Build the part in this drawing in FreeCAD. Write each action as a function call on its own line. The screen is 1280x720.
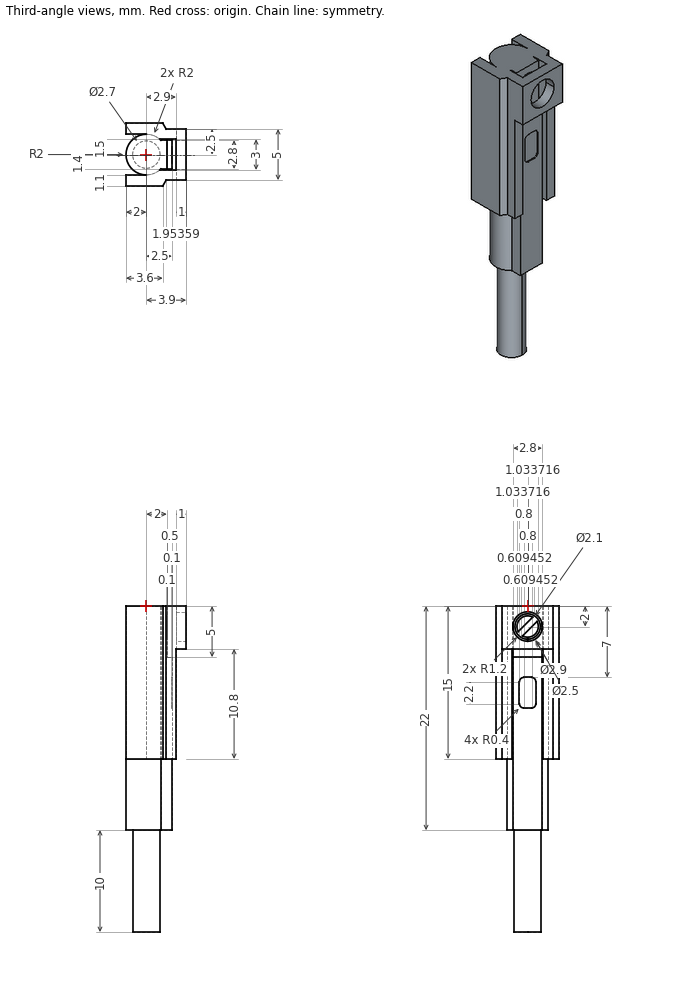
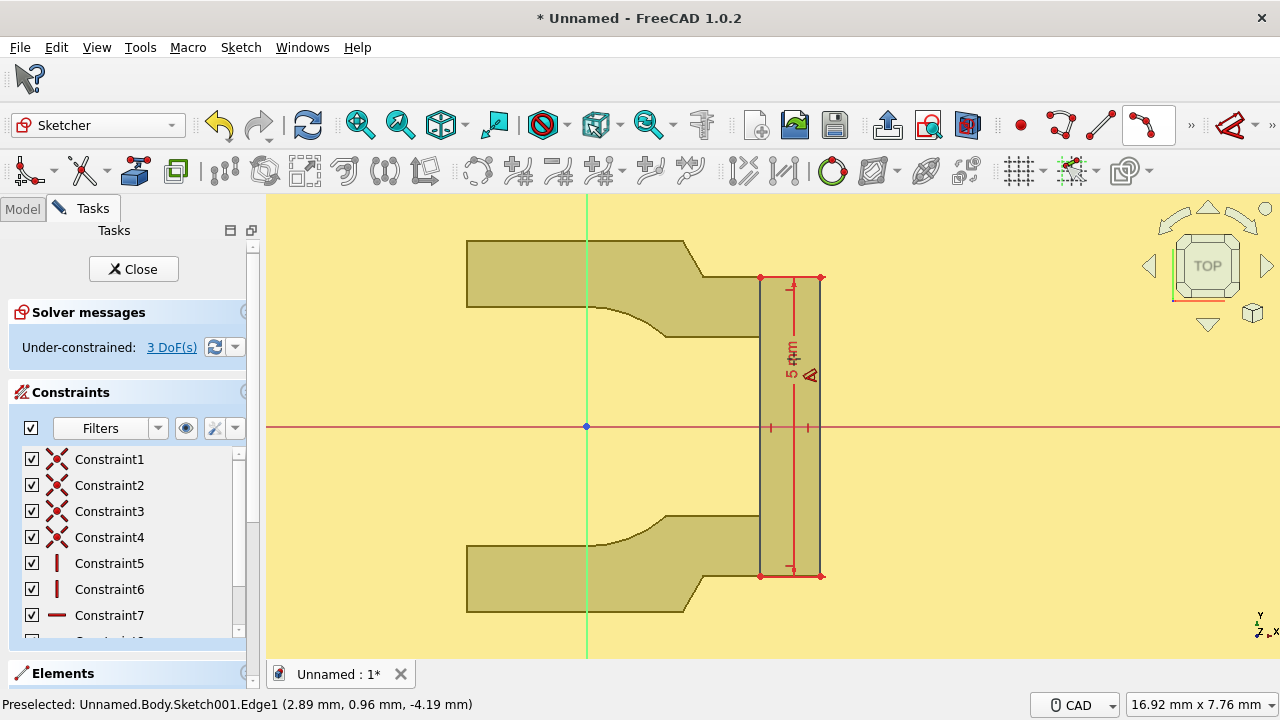
click(778, 577)
click(790, 611)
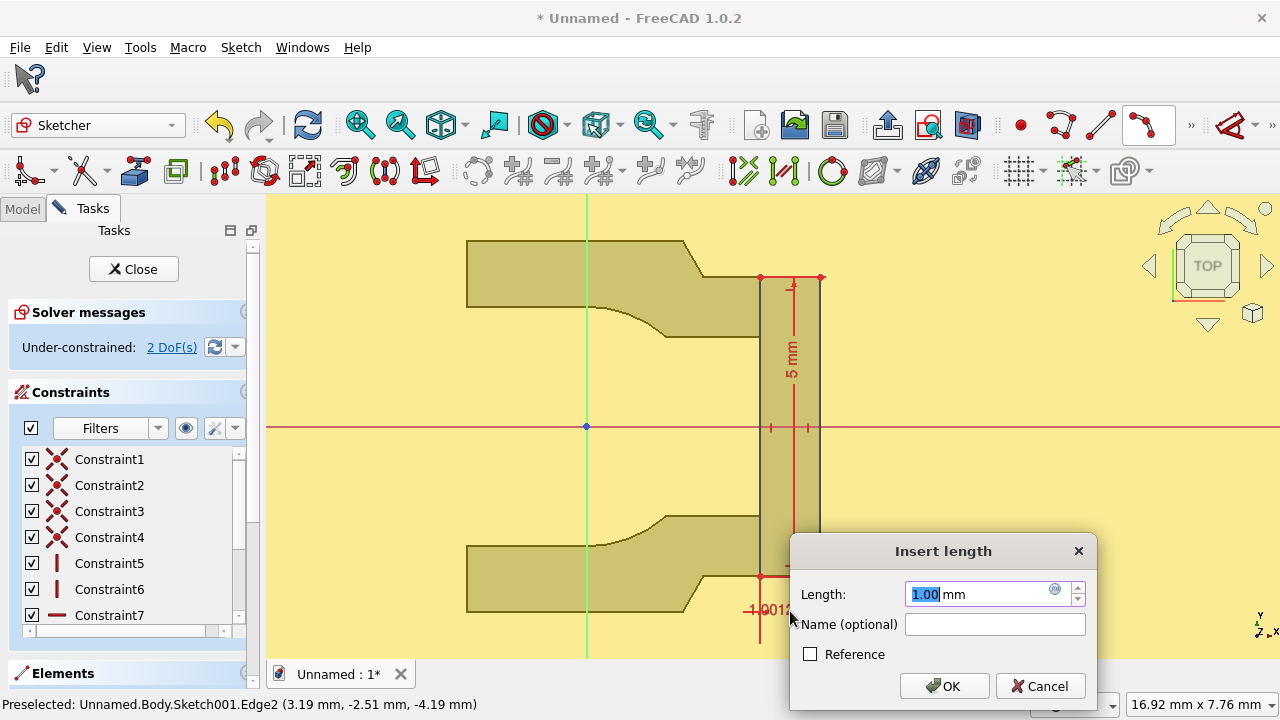
text(1)
key(Return)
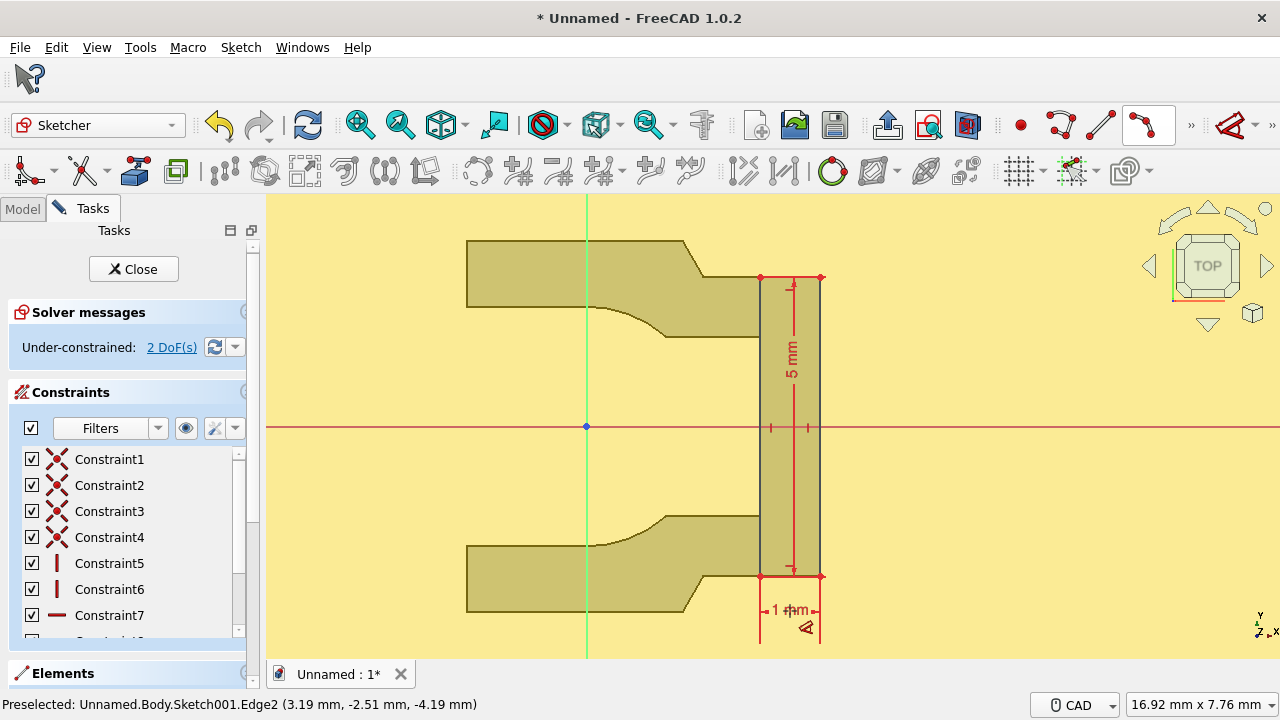
click(760, 277)
click(673, 243)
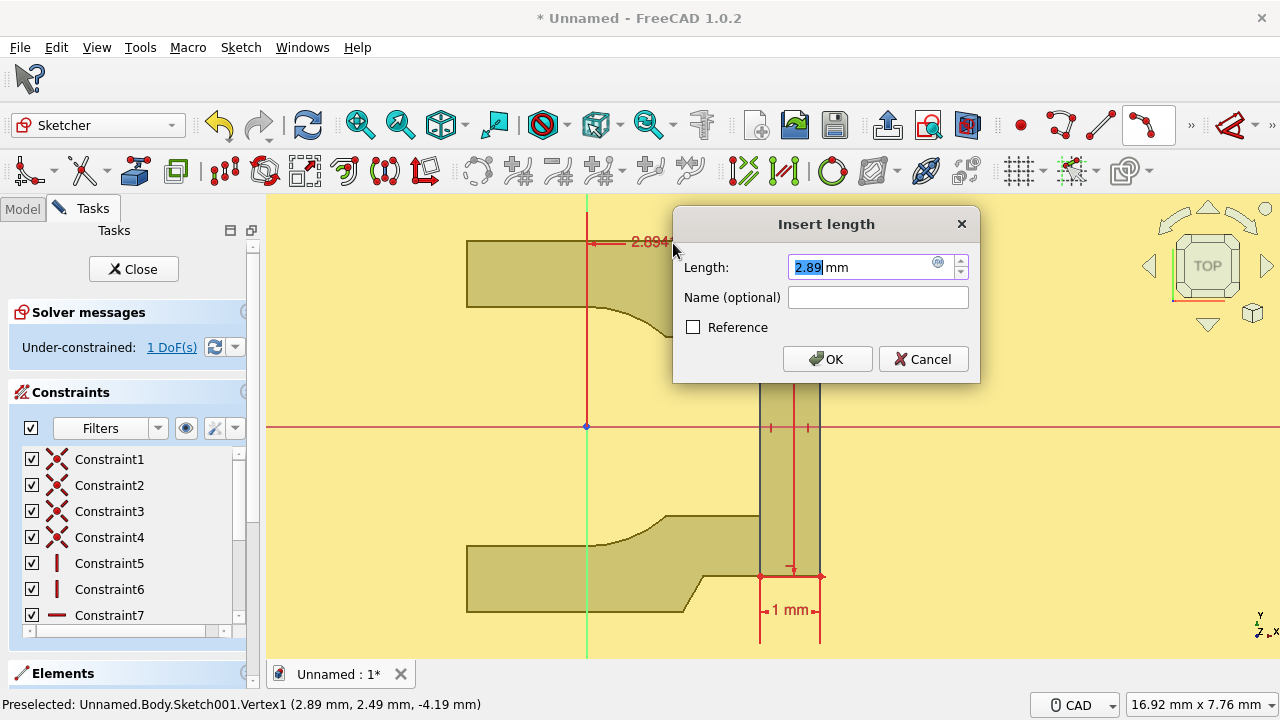
text(2.9)
key(Return)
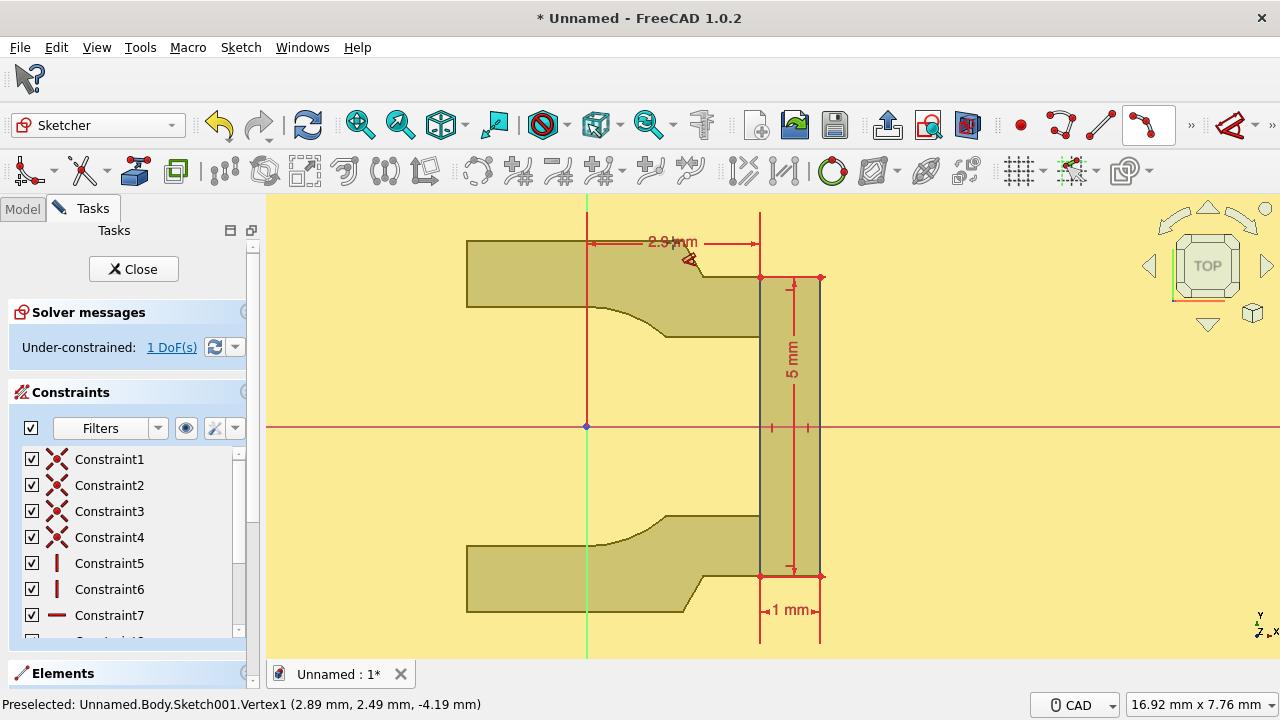
click(760, 277)
click(553, 352)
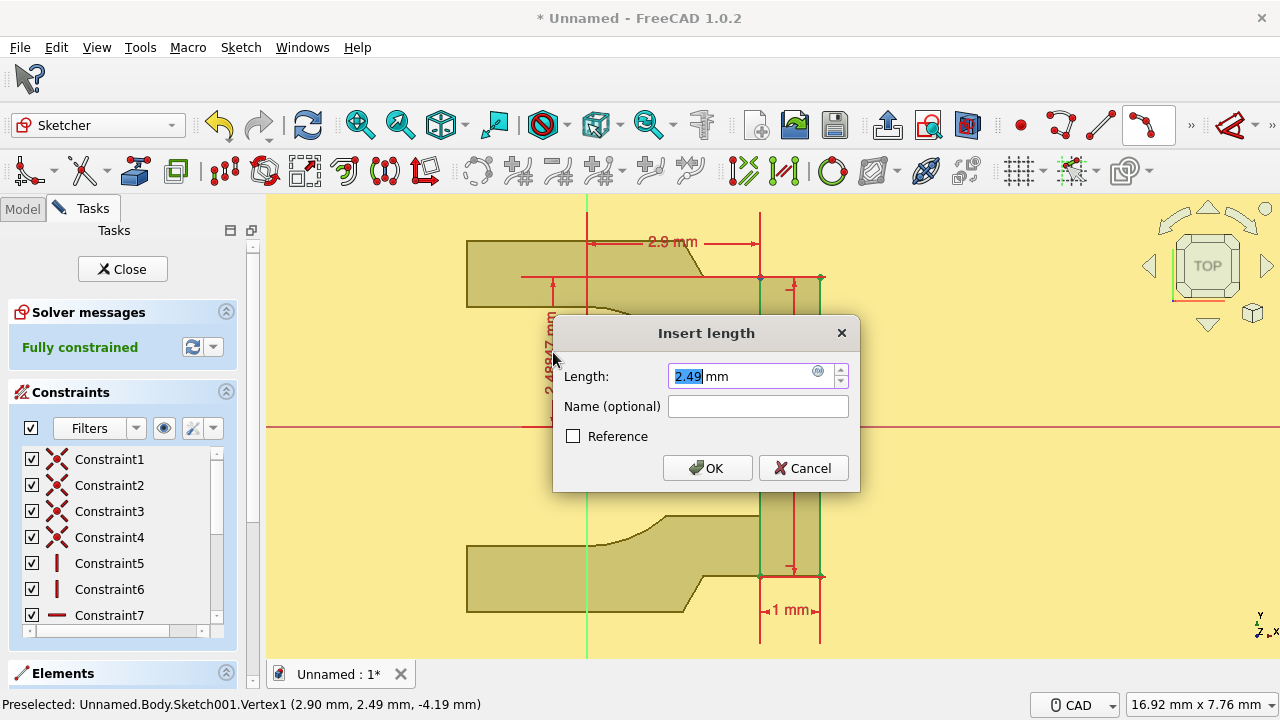
text(2.5)
key(Return)
key(Escape)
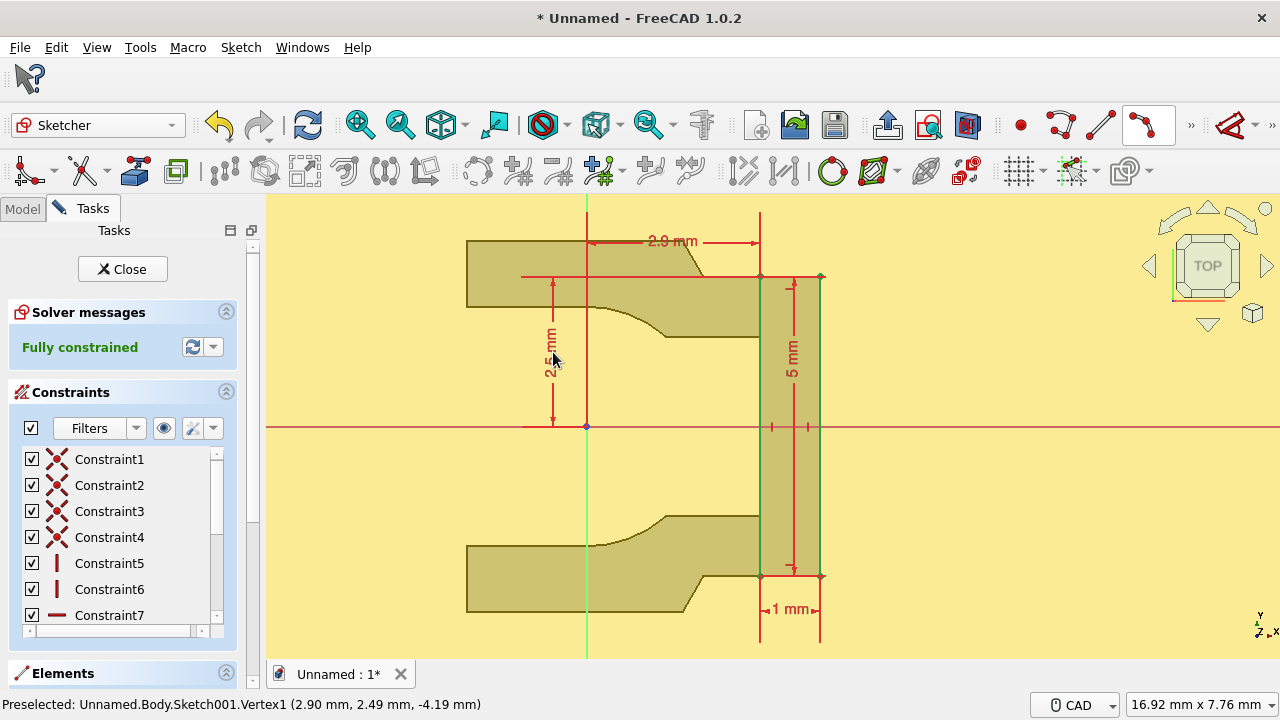
click(123, 269)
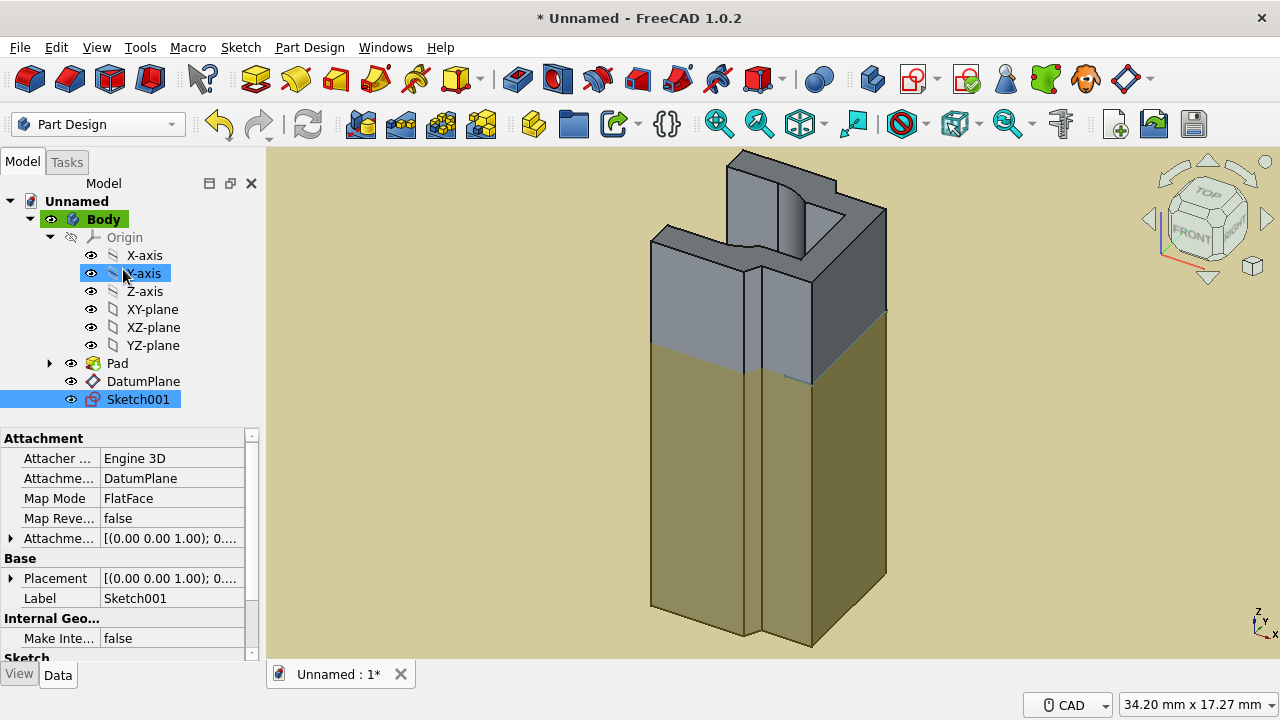
click(518, 80)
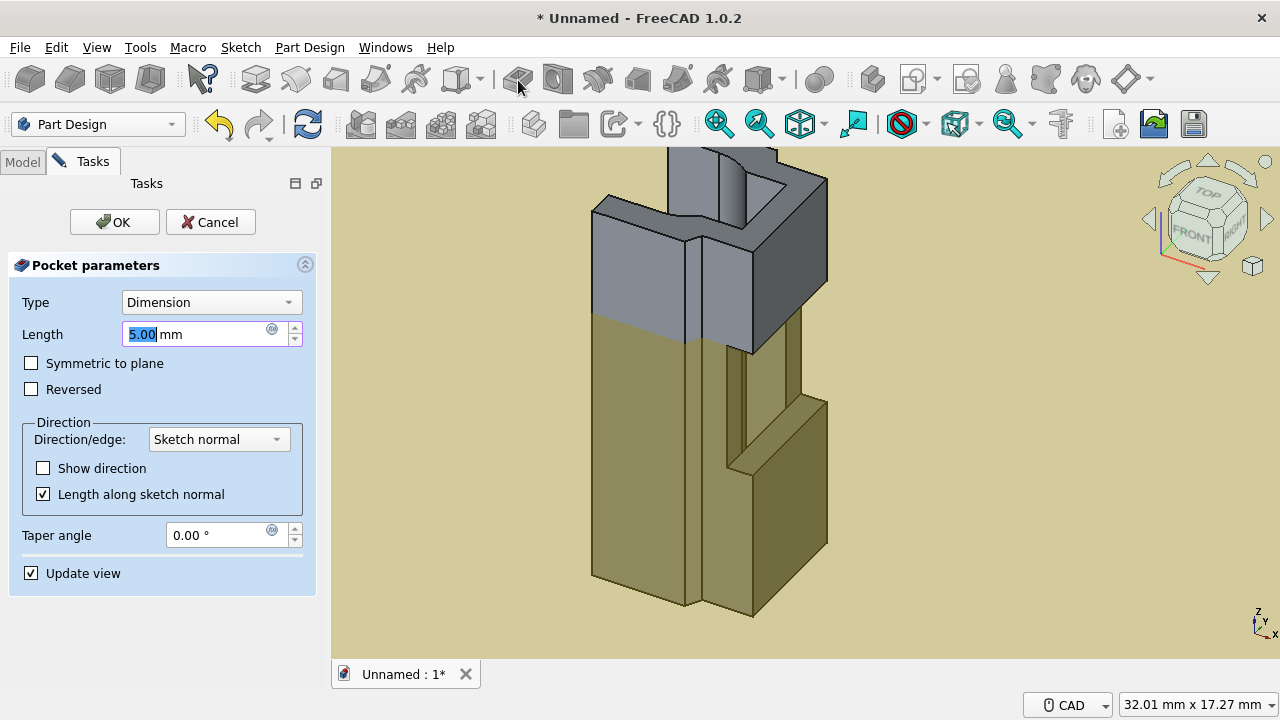
text(10.8)
key(Tab)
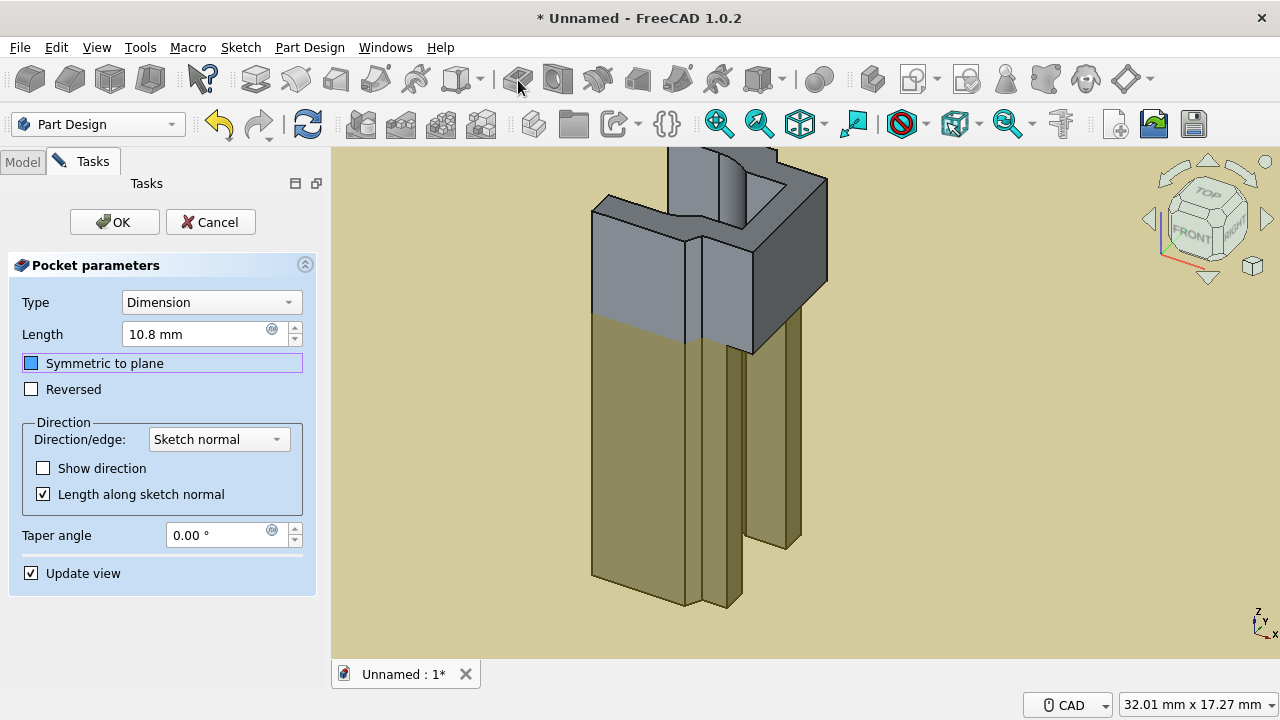
click(115, 222)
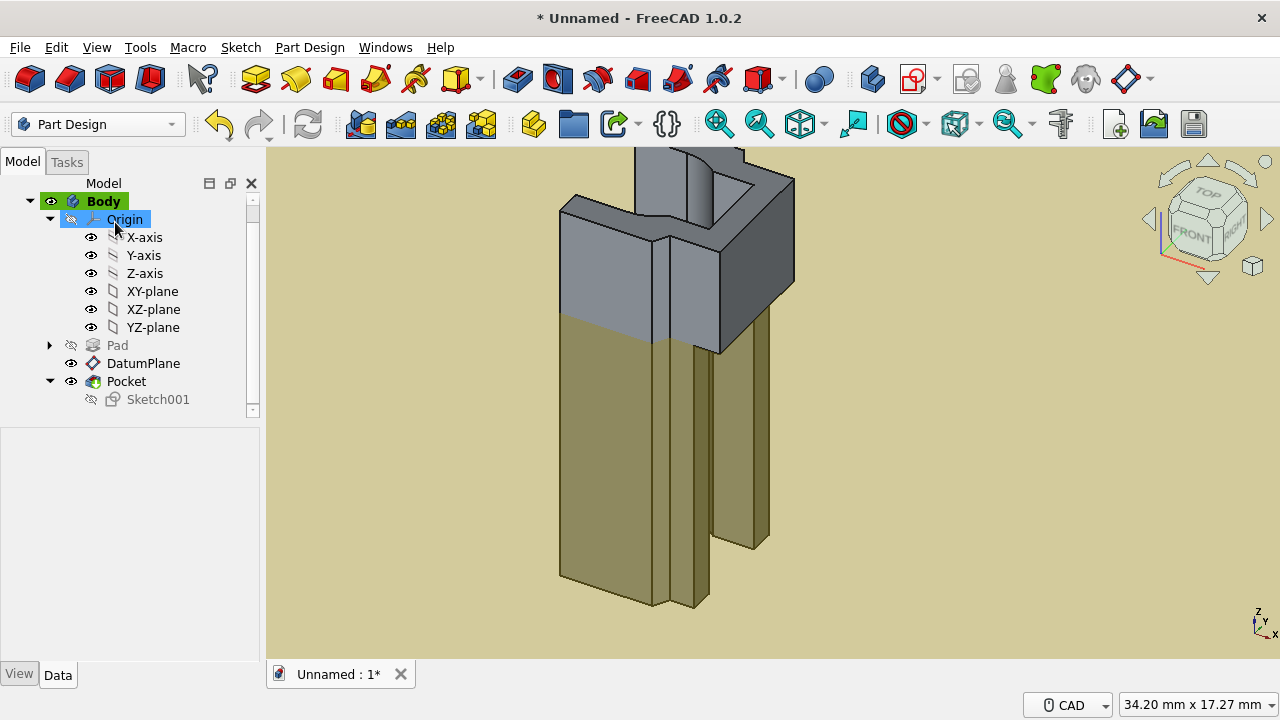
click(116, 363)
key(space)